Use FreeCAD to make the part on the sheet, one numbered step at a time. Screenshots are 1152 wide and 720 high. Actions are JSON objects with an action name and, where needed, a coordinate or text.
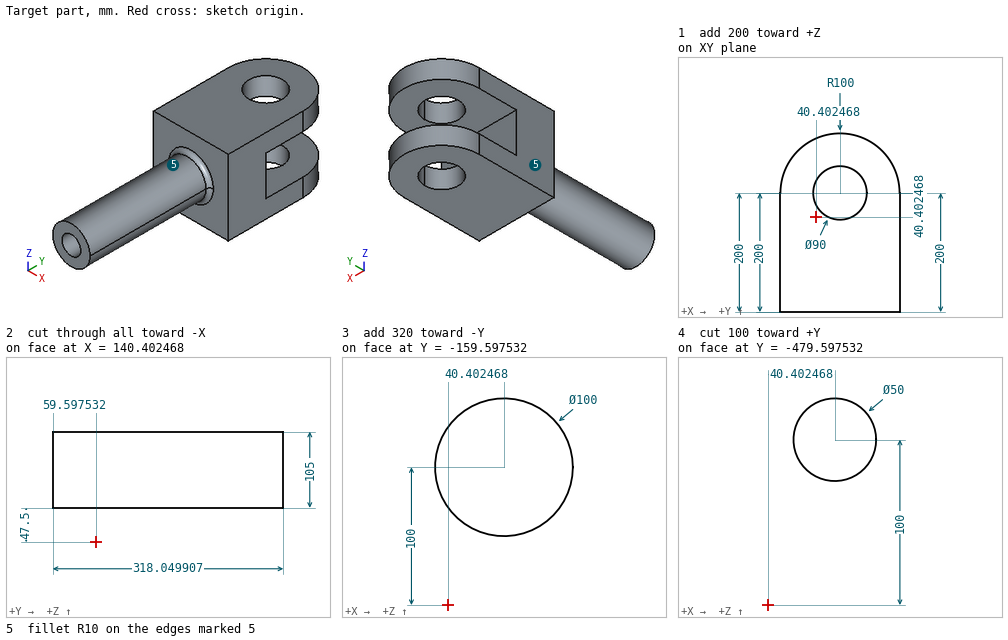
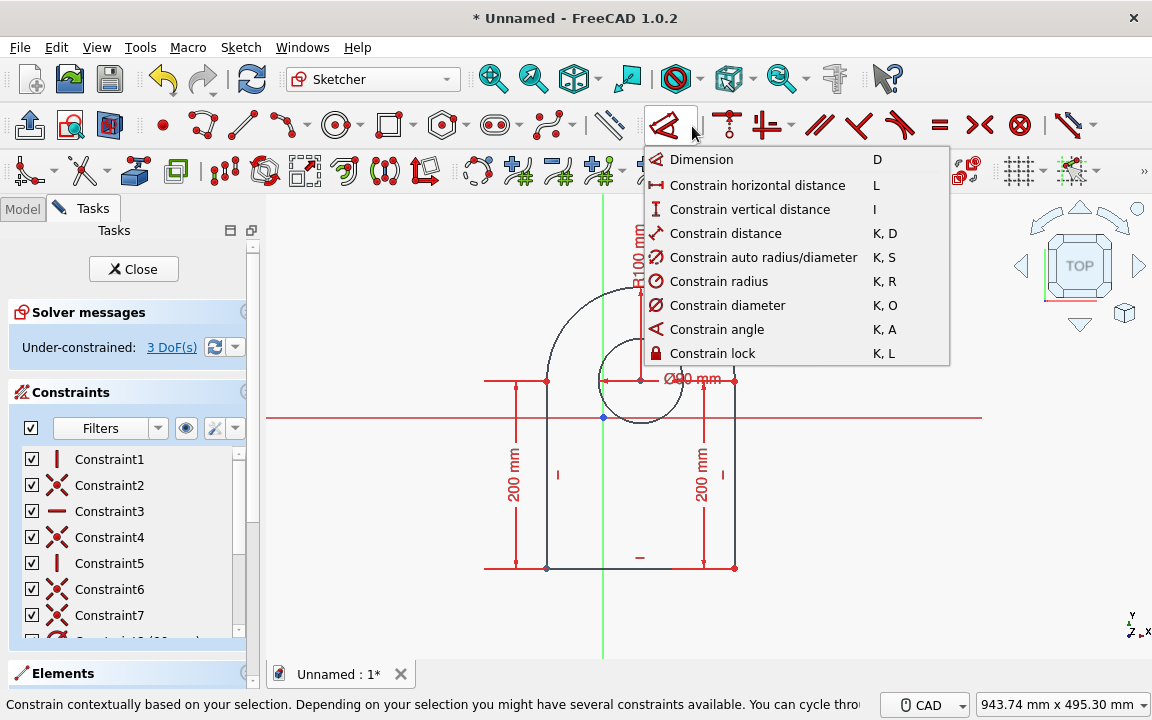
{"action": "left_click", "coordinate": [797, 209]}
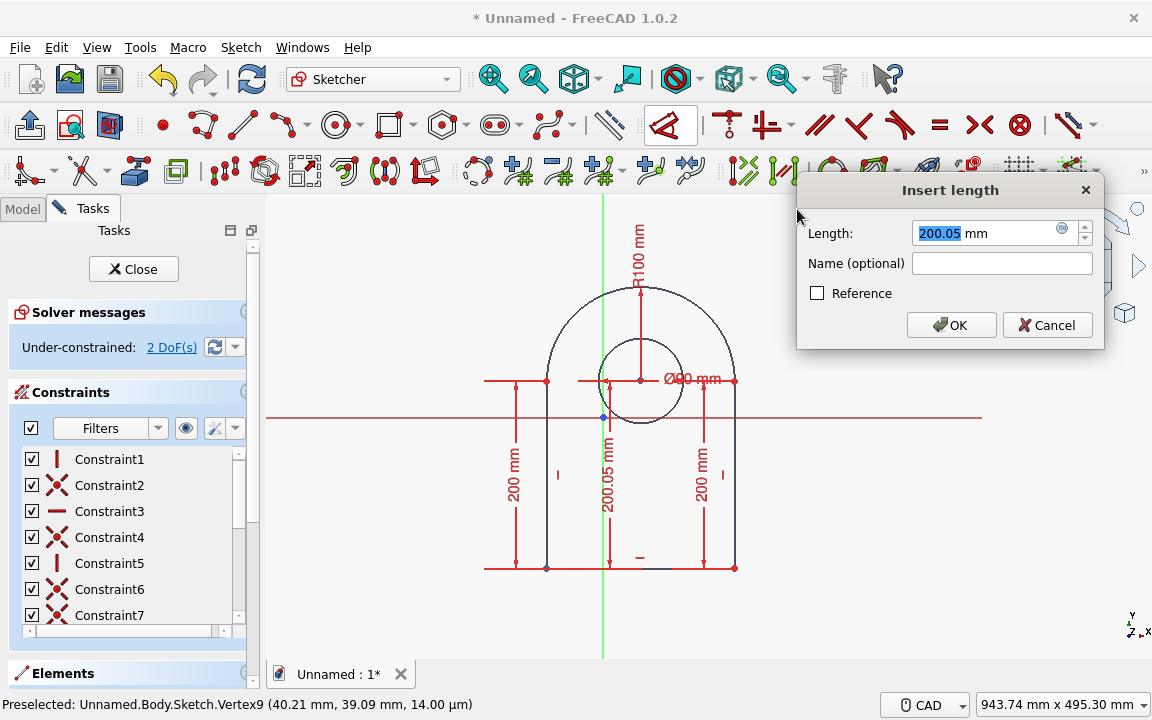
{"action": "type", "text": "200"}
{"action": "key", "text": "Return"}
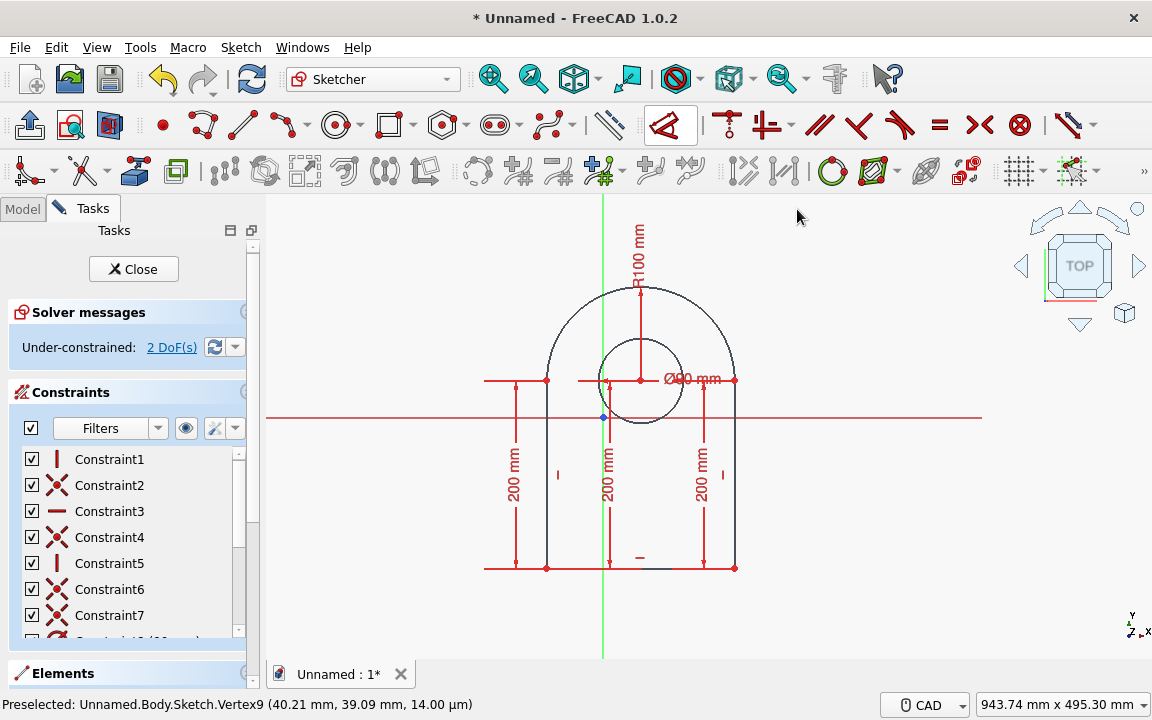
{"action": "left_click", "coordinate": [641, 381]}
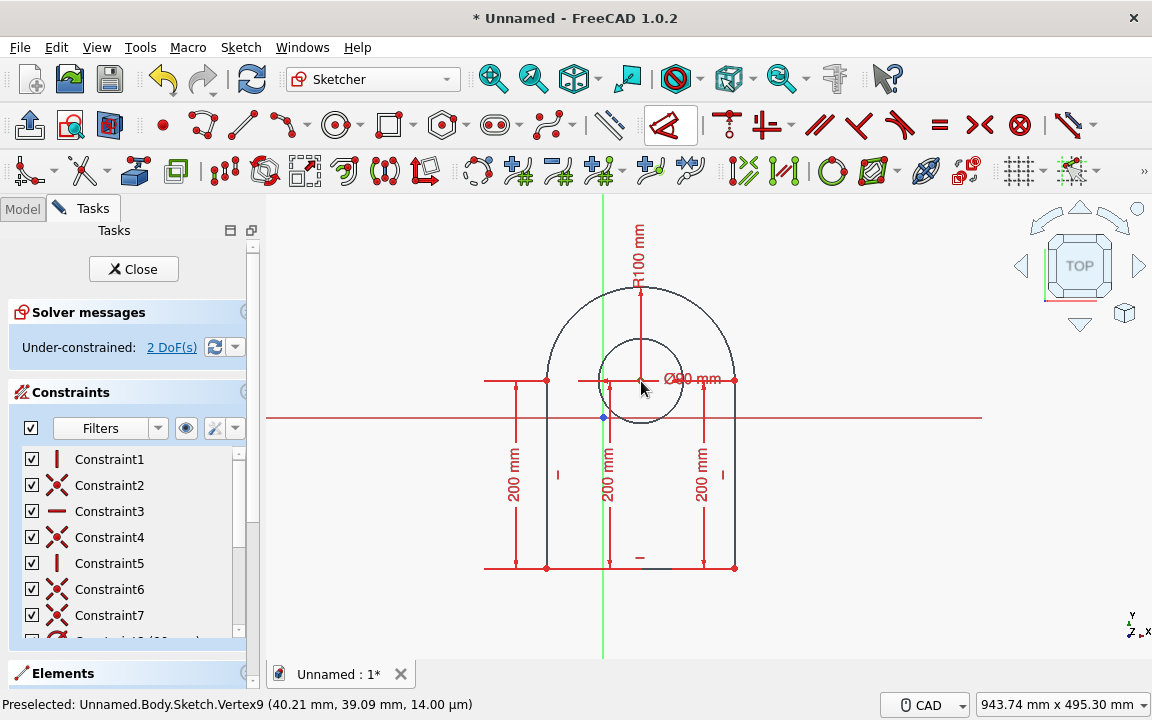
{"action": "key", "text": "l"}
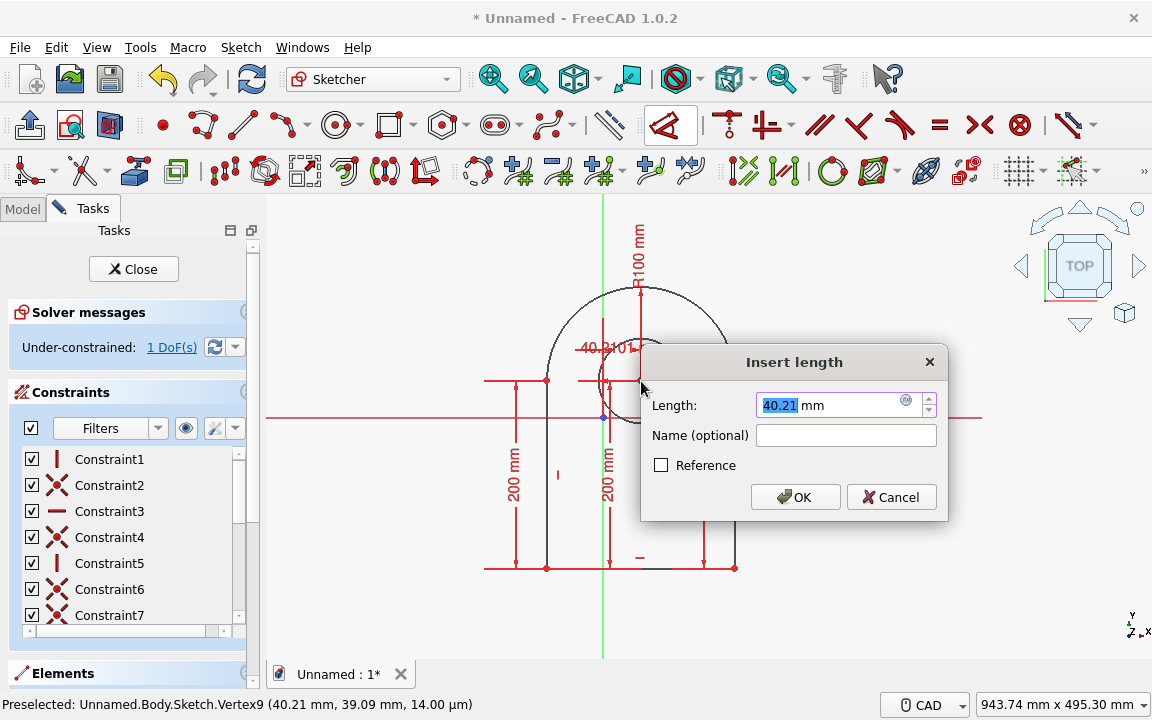
{"action": "type", "text": "40.402468"}
{"action": "key", "text": "Return"}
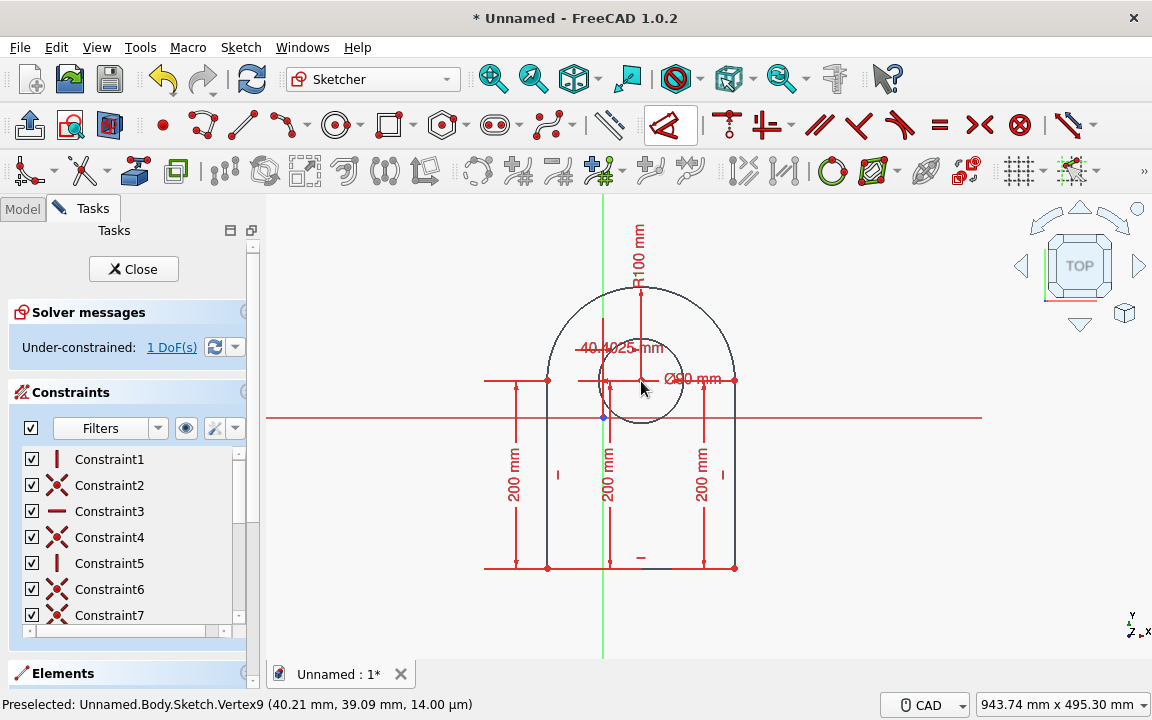
{"action": "left_click", "coordinate": [641, 381]}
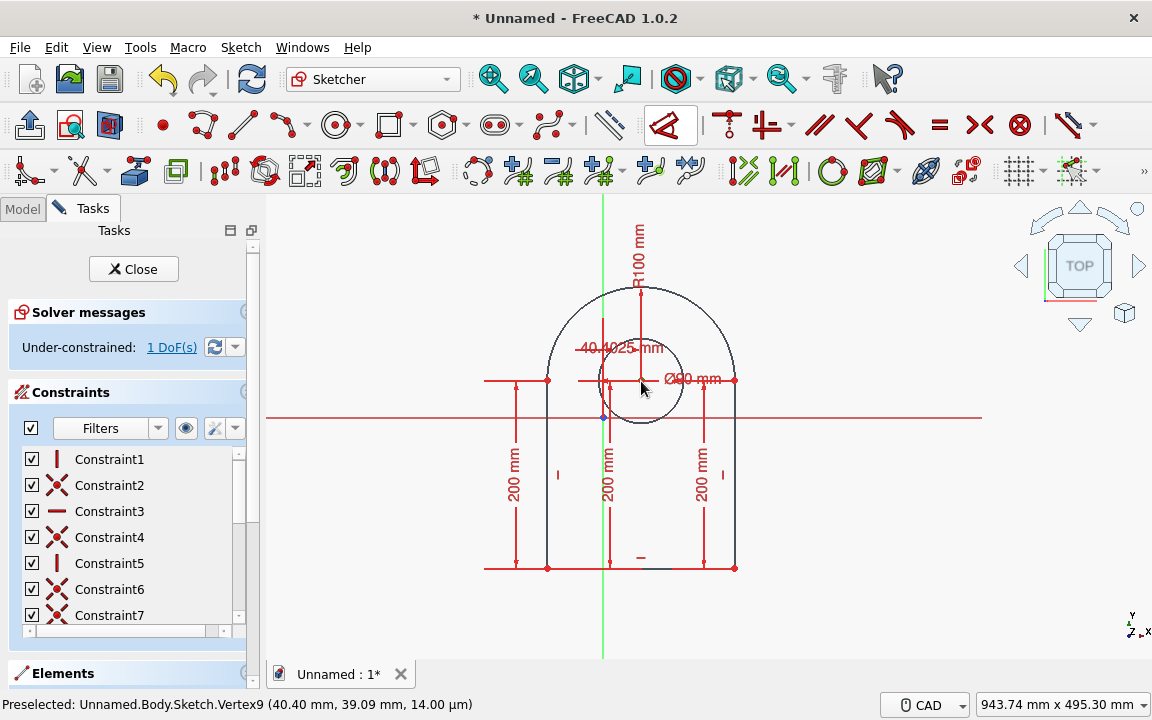
{"action": "left_click", "coordinate": [692, 126]}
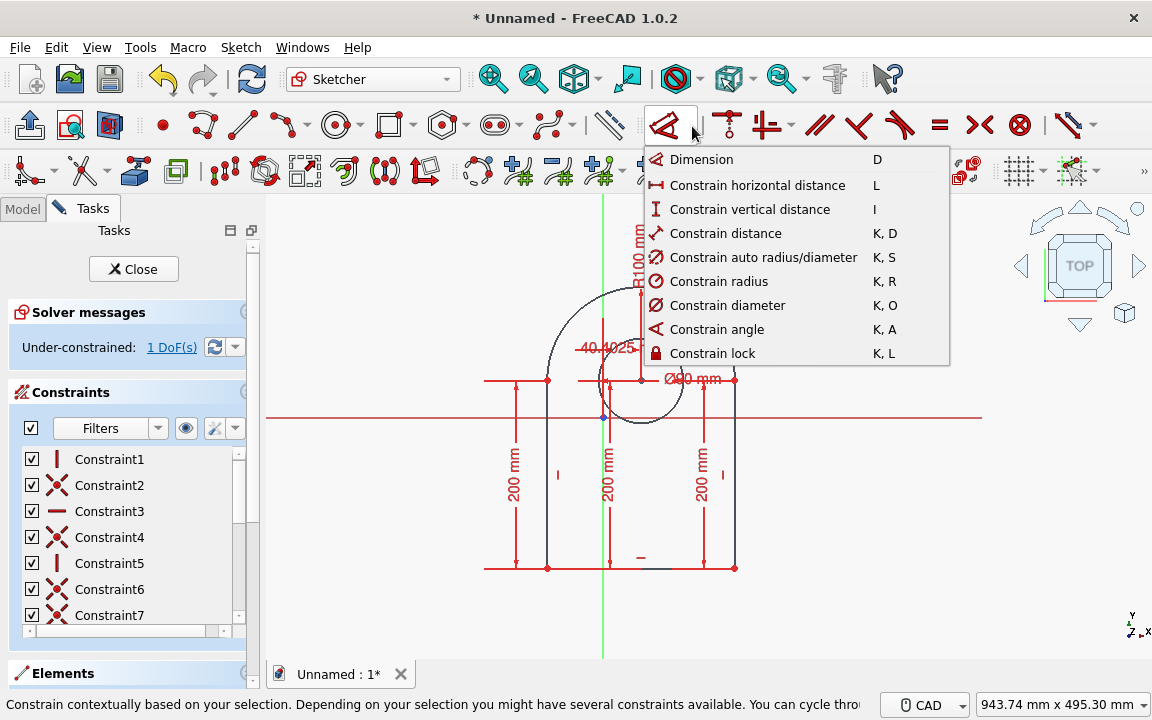
{"action": "left_click", "coordinate": [797, 209]}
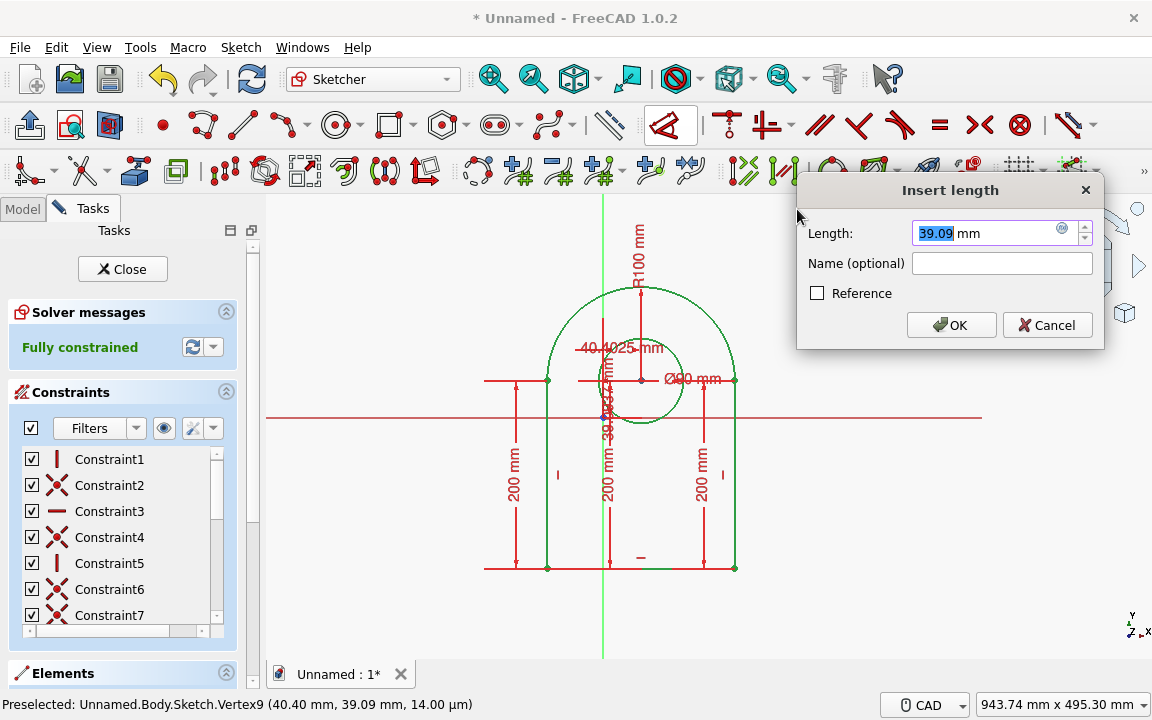
{"action": "type", "text": "40.402468"}
{"action": "key", "text": "Return"}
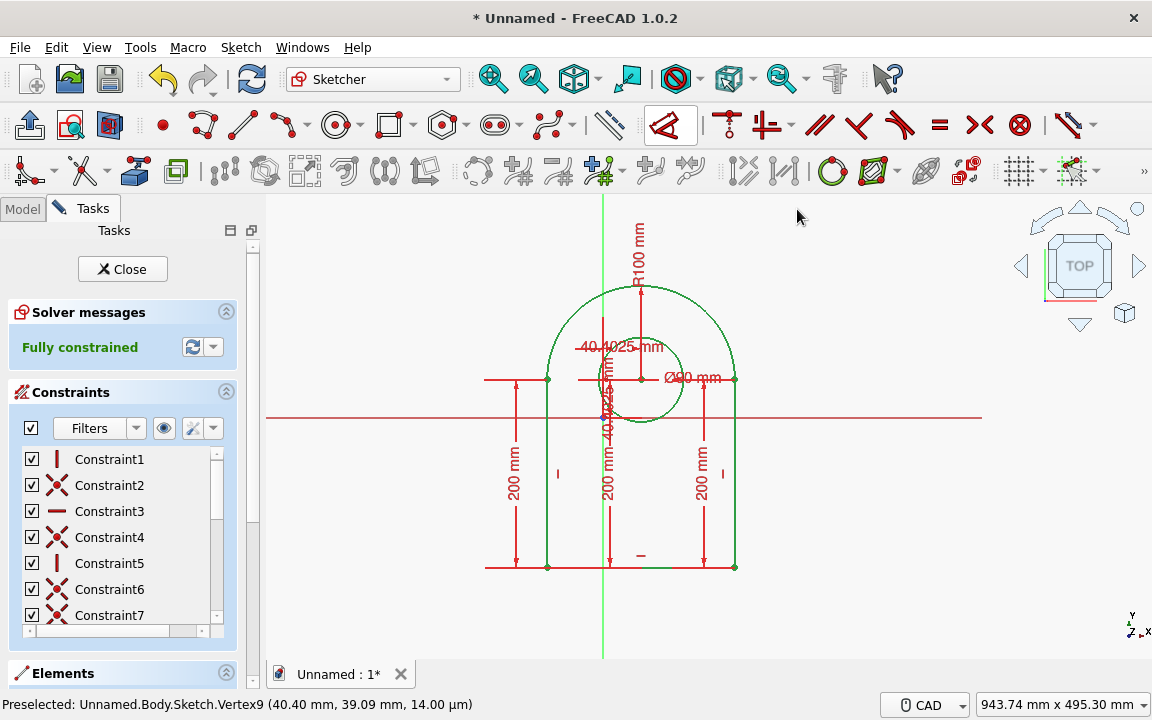
{"action": "left_click", "coordinate": [123, 269]}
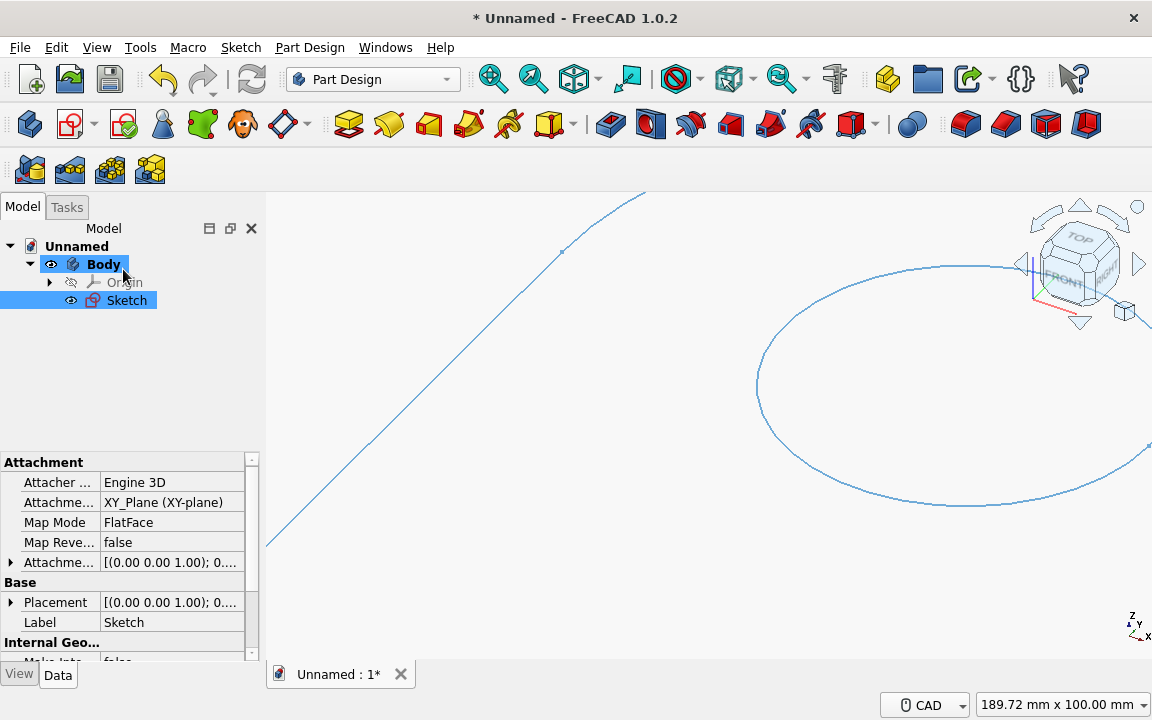
{"action": "left_click", "coordinate": [350, 124]}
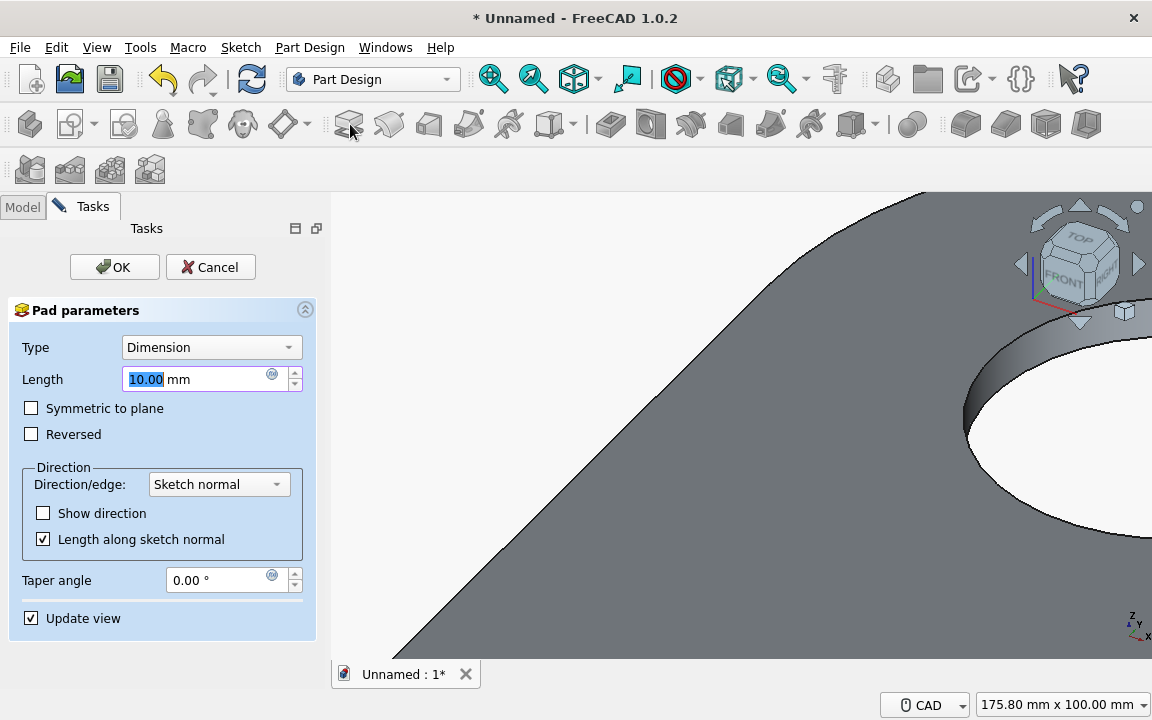
{"action": "type", "text": "200"}
{"action": "key", "text": "Tab"}